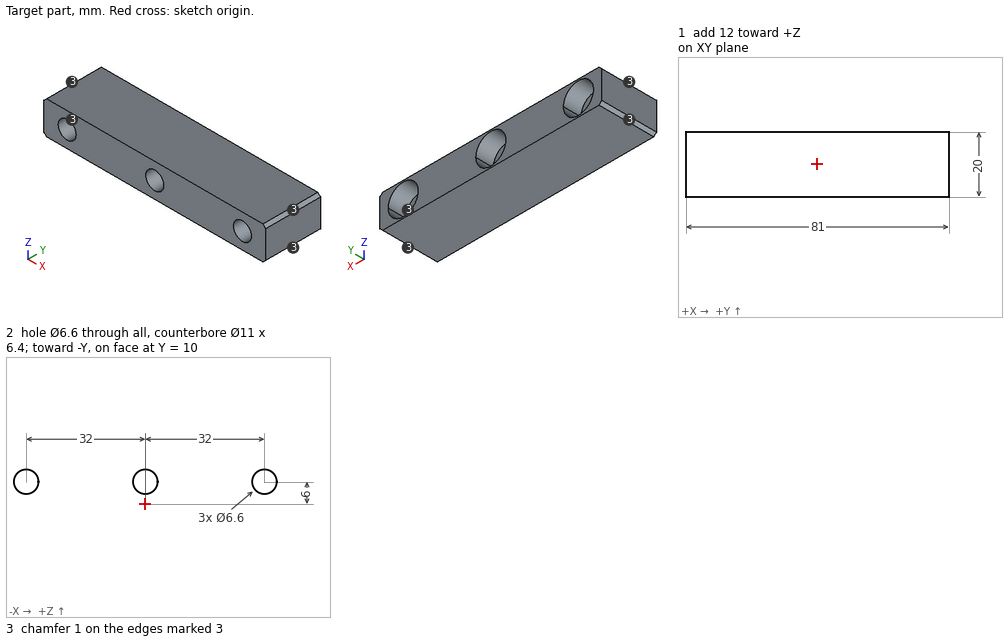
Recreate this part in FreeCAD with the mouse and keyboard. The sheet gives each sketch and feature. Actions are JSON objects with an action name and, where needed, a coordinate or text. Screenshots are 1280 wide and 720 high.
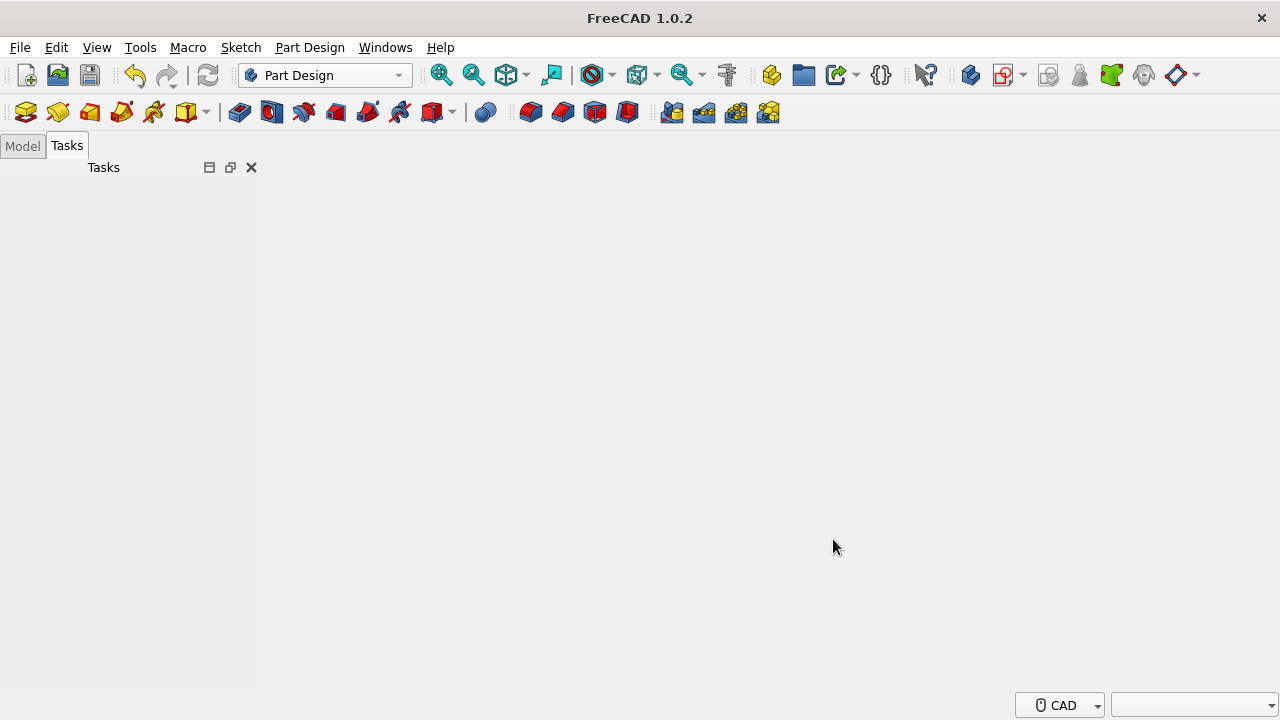
{"action": "left_click", "coordinate": [26, 76]}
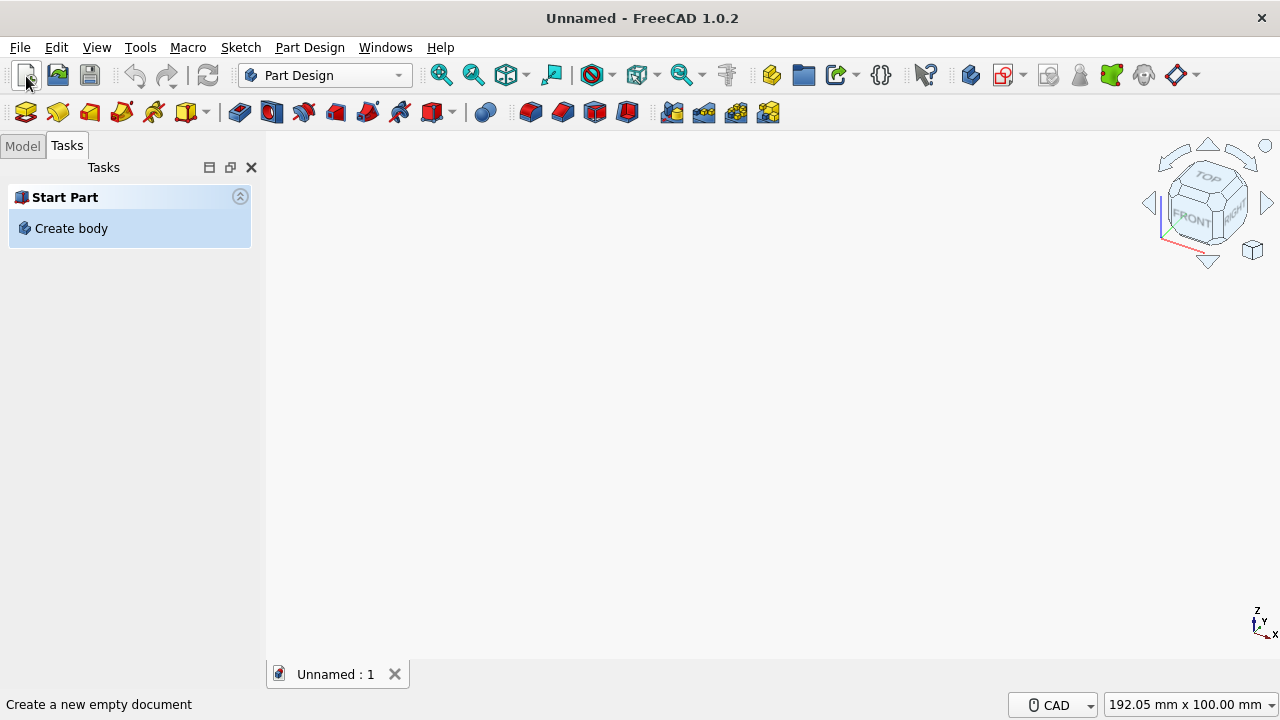
{"action": "left_click", "coordinate": [1004, 76]}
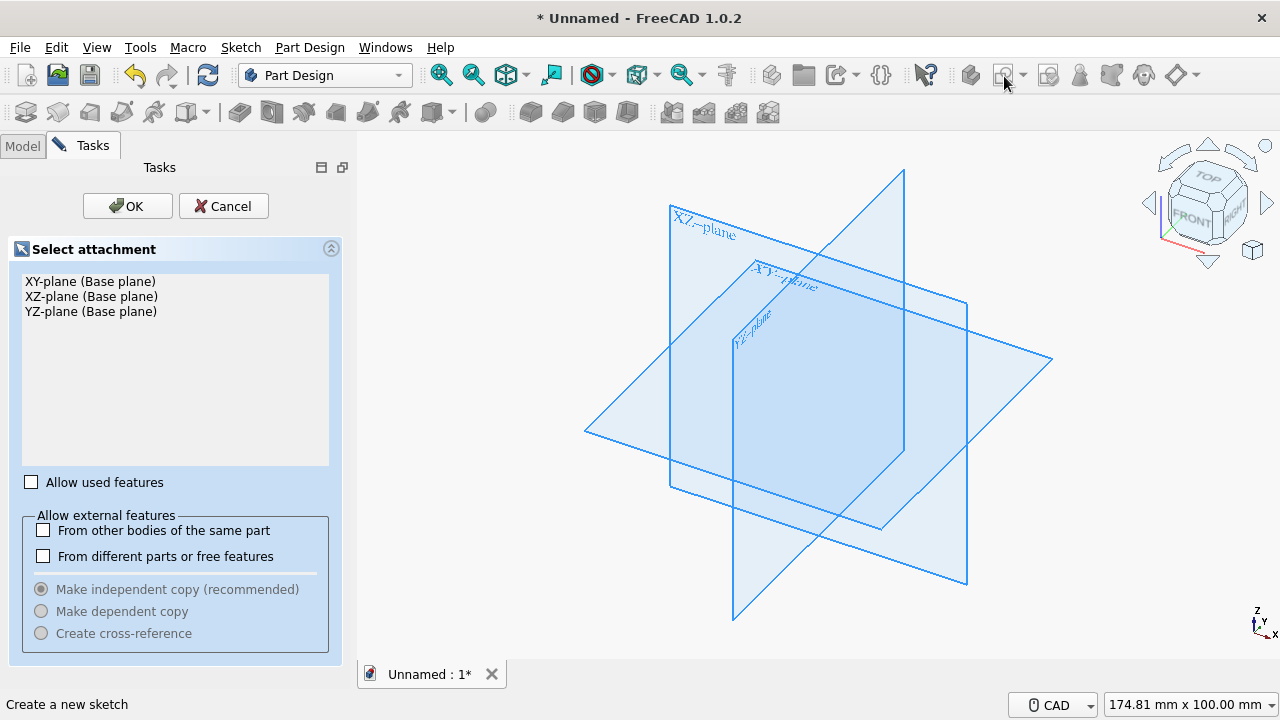
{"action": "left_click", "coordinate": [82, 282]}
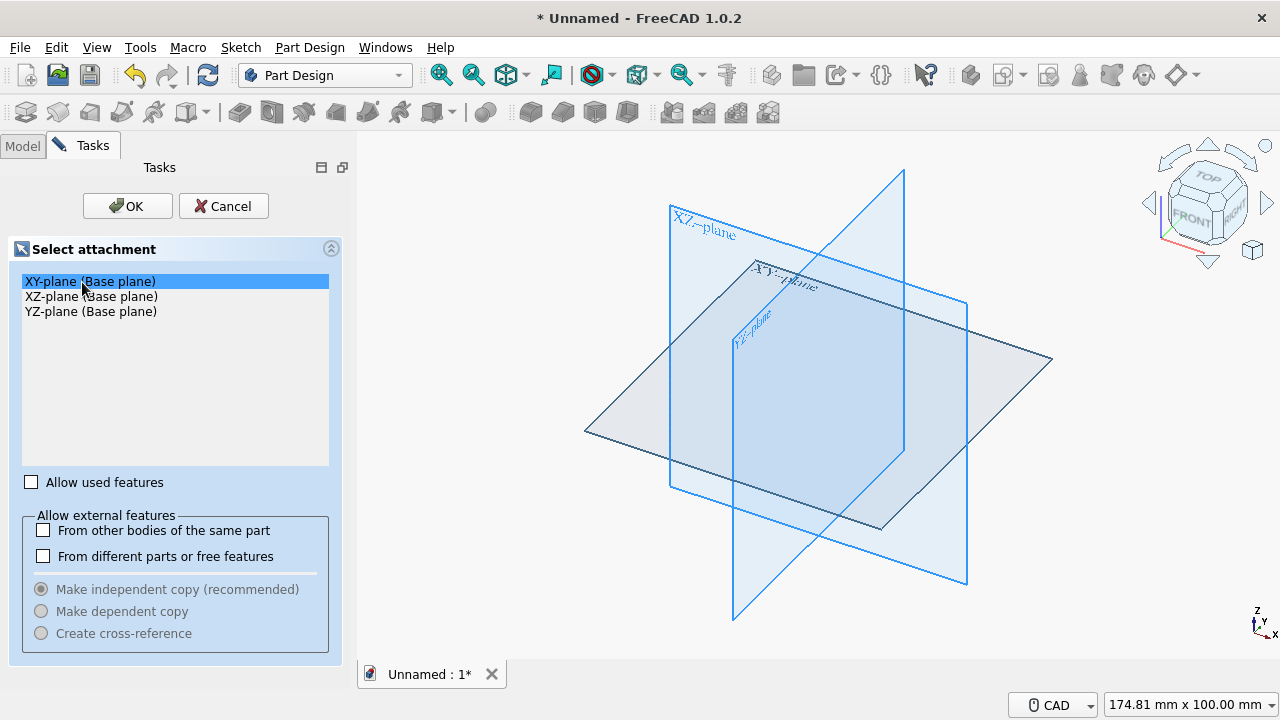
{"action": "left_click", "coordinate": [128, 206]}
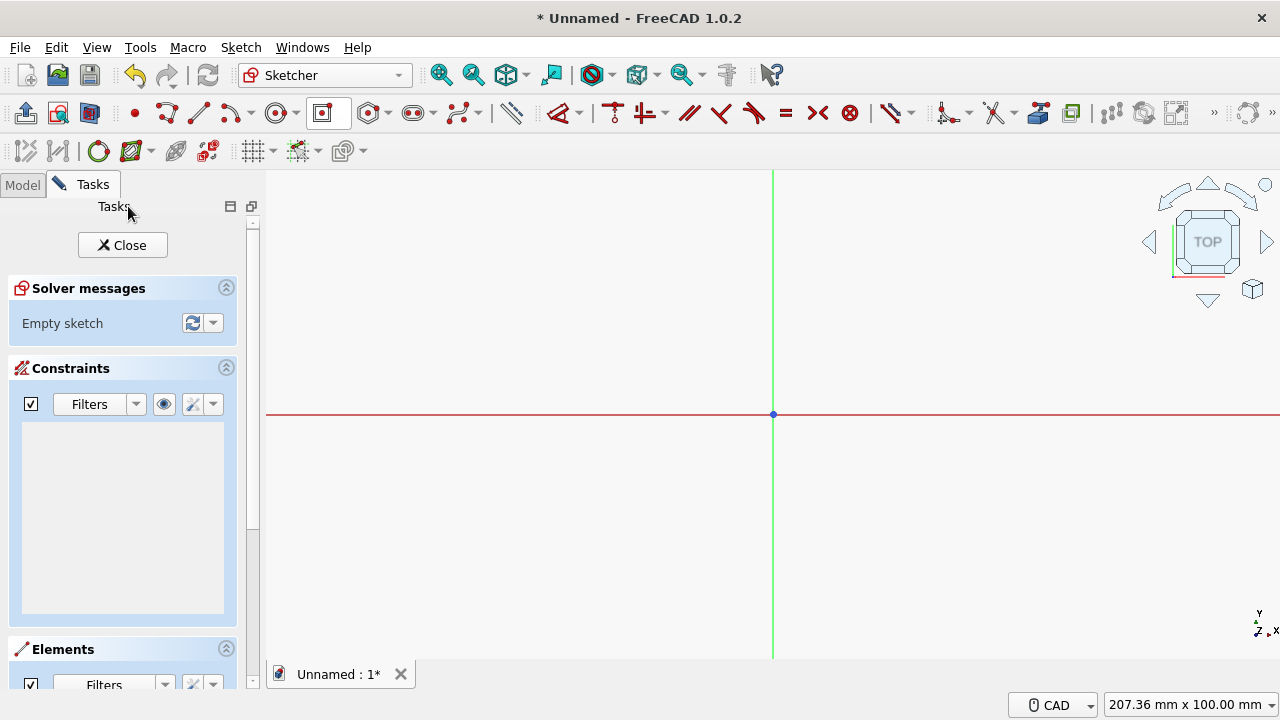
{"action": "scroll", "coordinate": [912, 414], "scroll_direction": "up", "scroll_amount": 2}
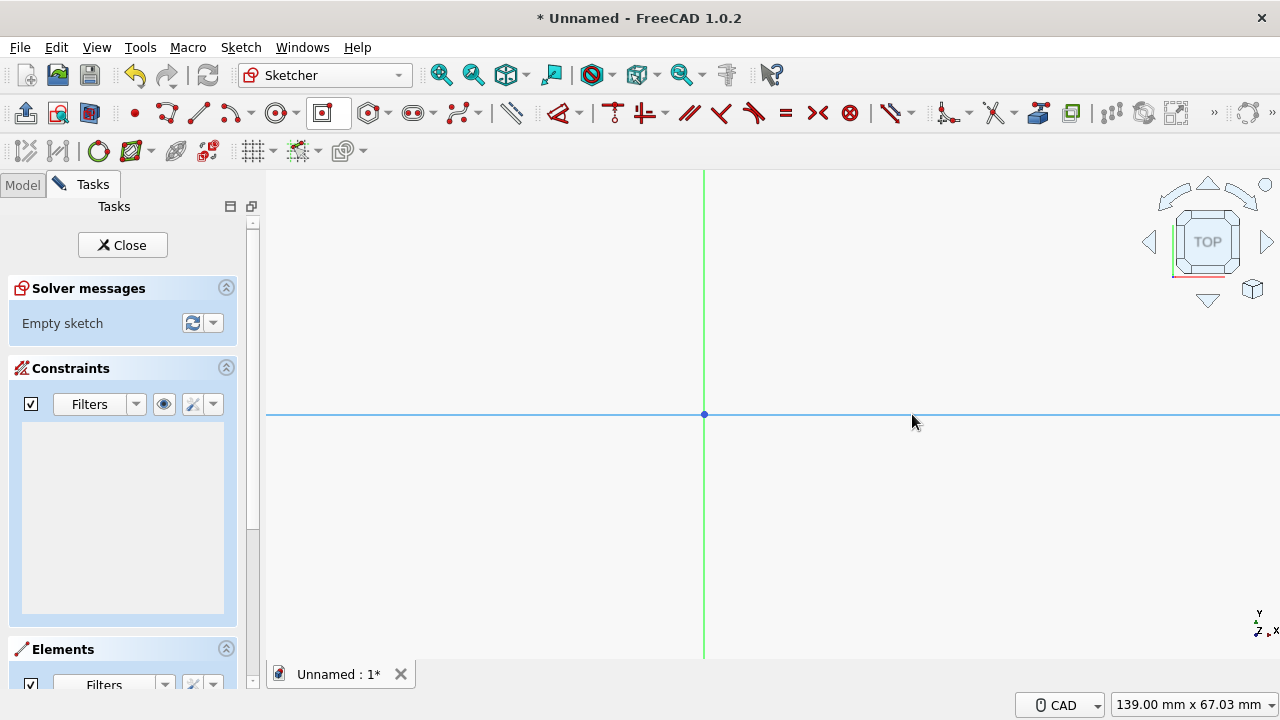
{"action": "left_click", "coordinate": [322, 114]}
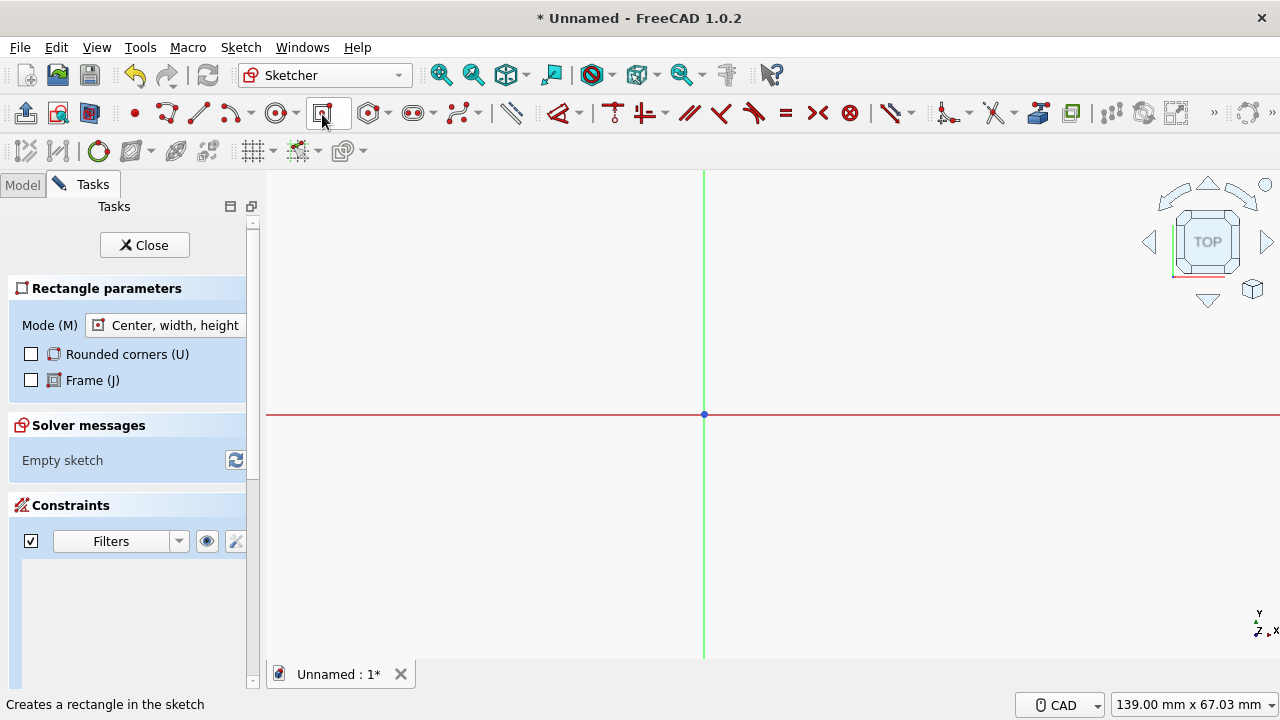
{"action": "left_click", "coordinate": [704, 414]}
{"action": "mouse_move", "coordinate": [1000, 342]}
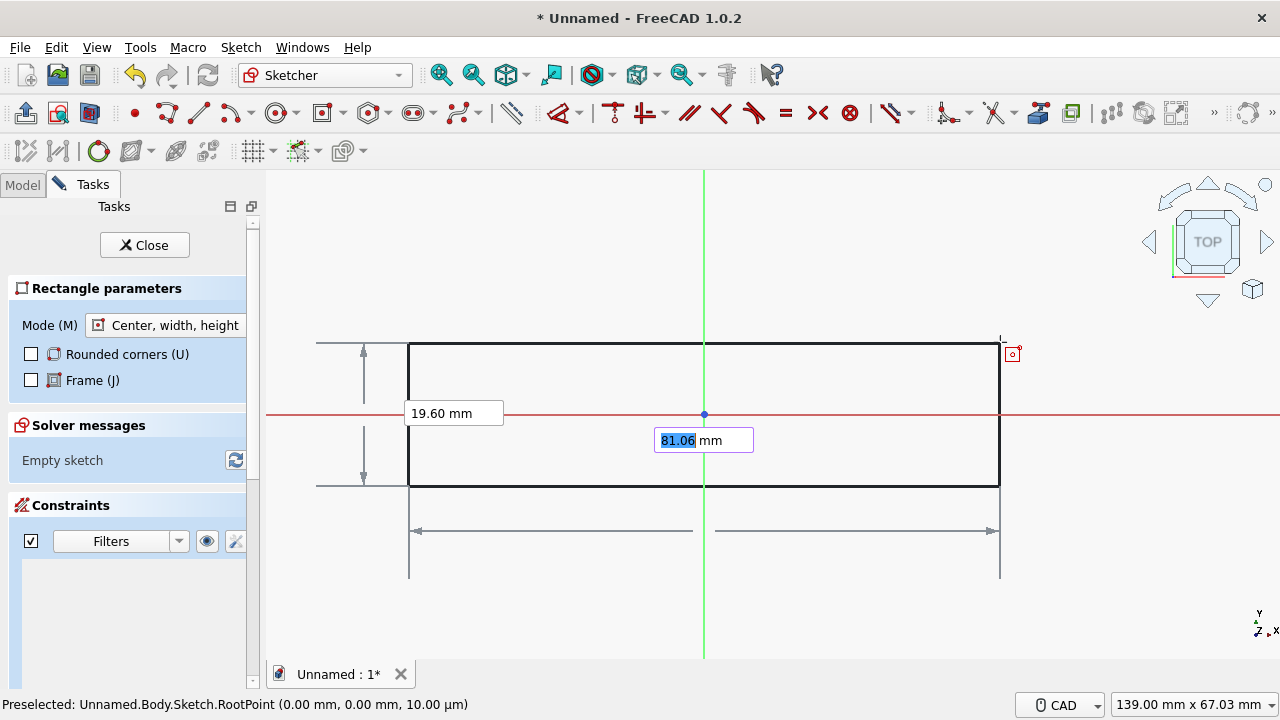
{"action": "type", "text": "81"}
{"action": "key", "text": "Tab"}
{"action": "type", "text": "20"}
{"action": "key", "text": "Return"}
{"action": "key", "text": "Escape"}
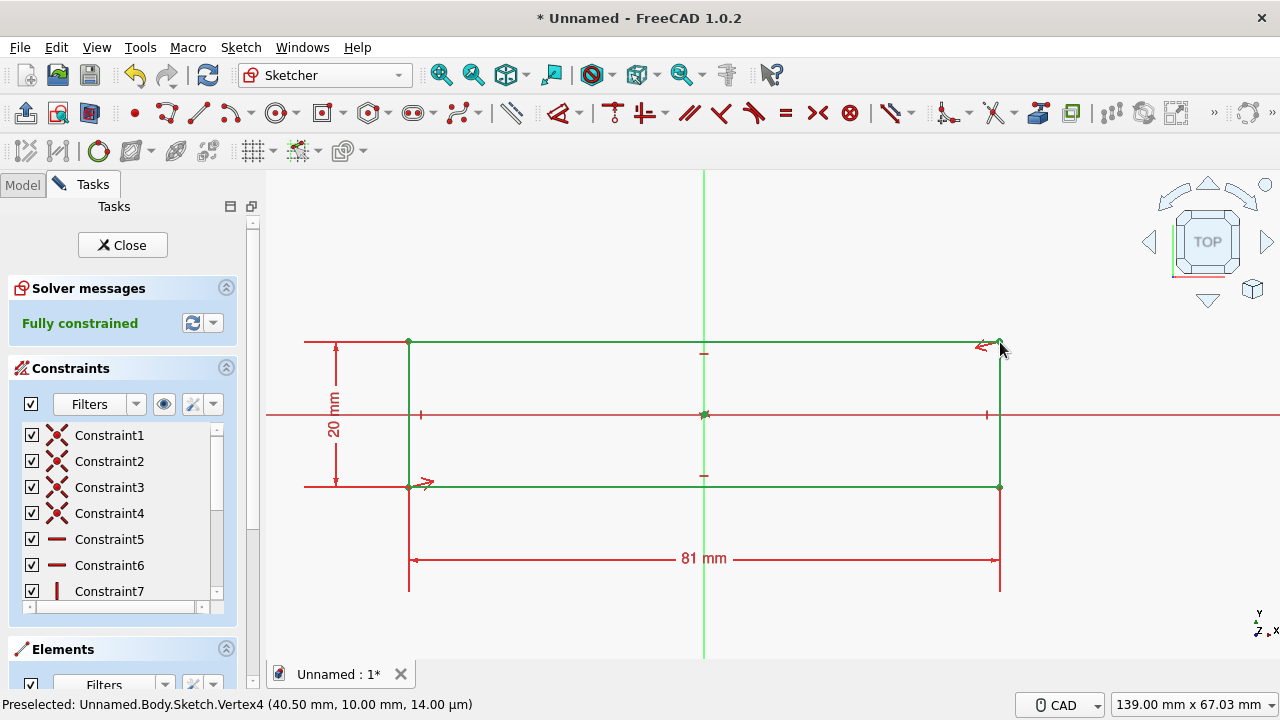
{"action": "left_click", "coordinate": [123, 245]}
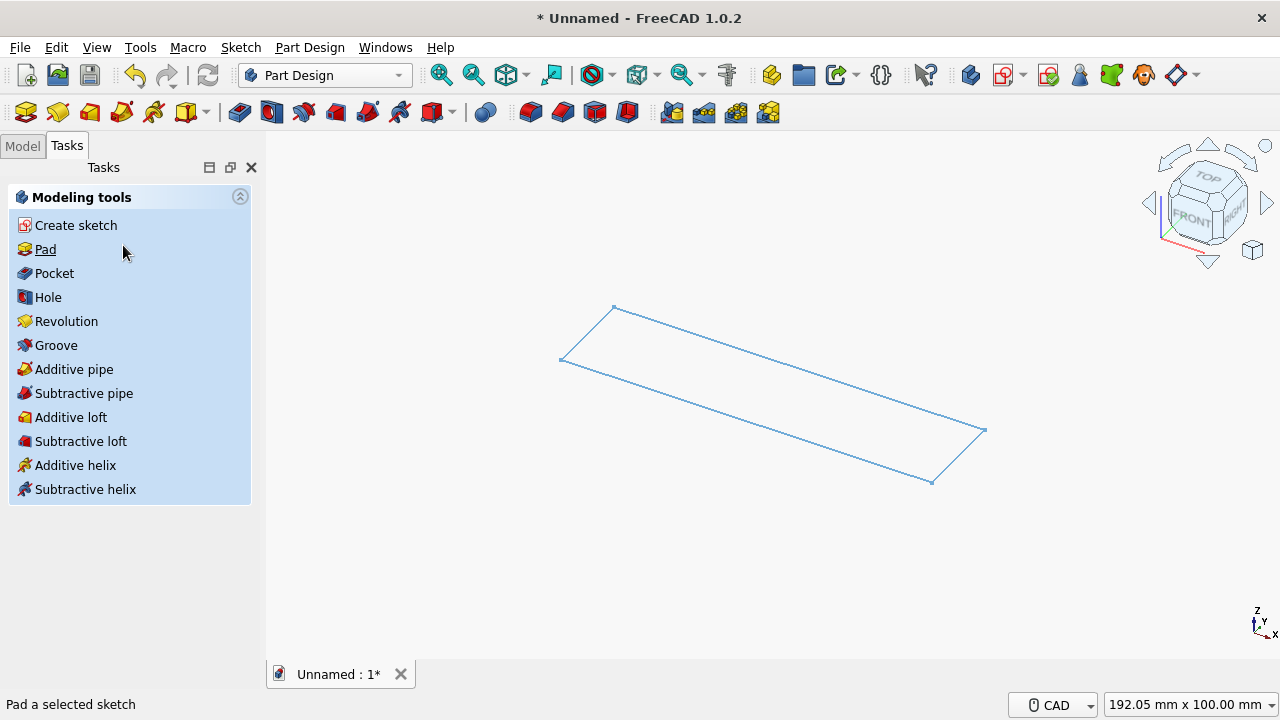
{"action": "left_click", "coordinate": [26, 112]}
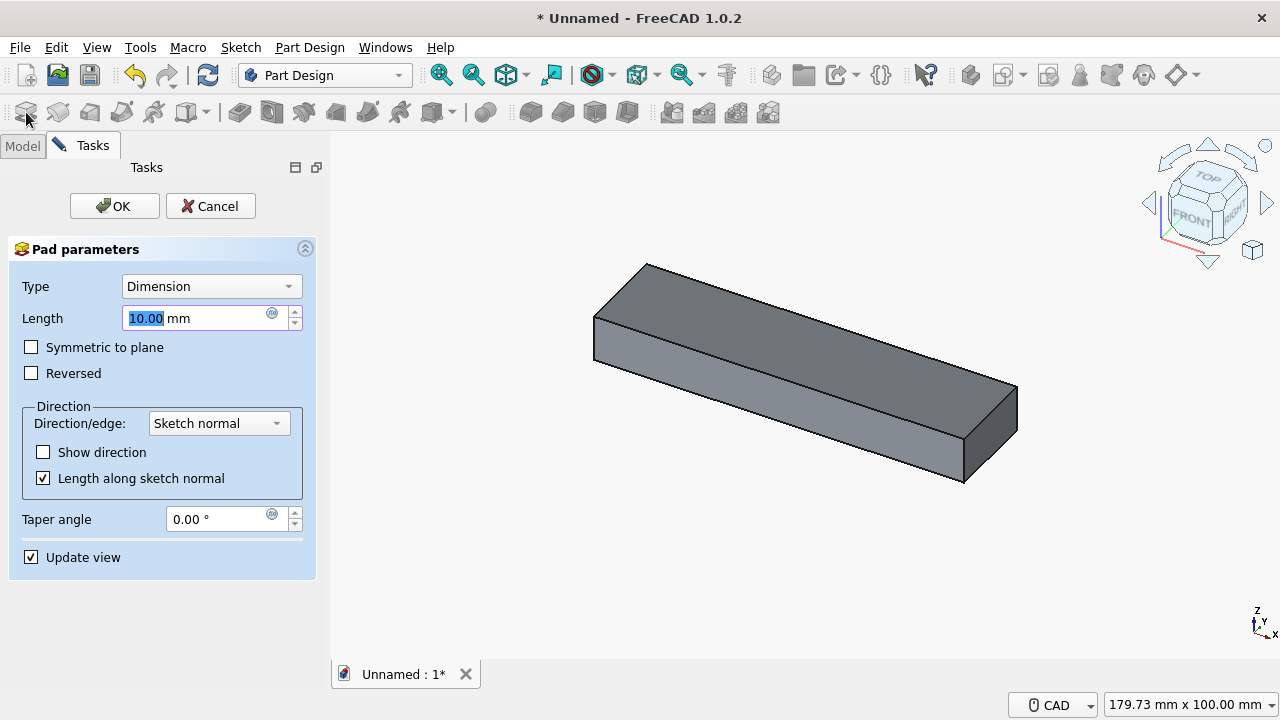
{"action": "type", "text": "12"}
{"action": "key", "text": "Tab"}